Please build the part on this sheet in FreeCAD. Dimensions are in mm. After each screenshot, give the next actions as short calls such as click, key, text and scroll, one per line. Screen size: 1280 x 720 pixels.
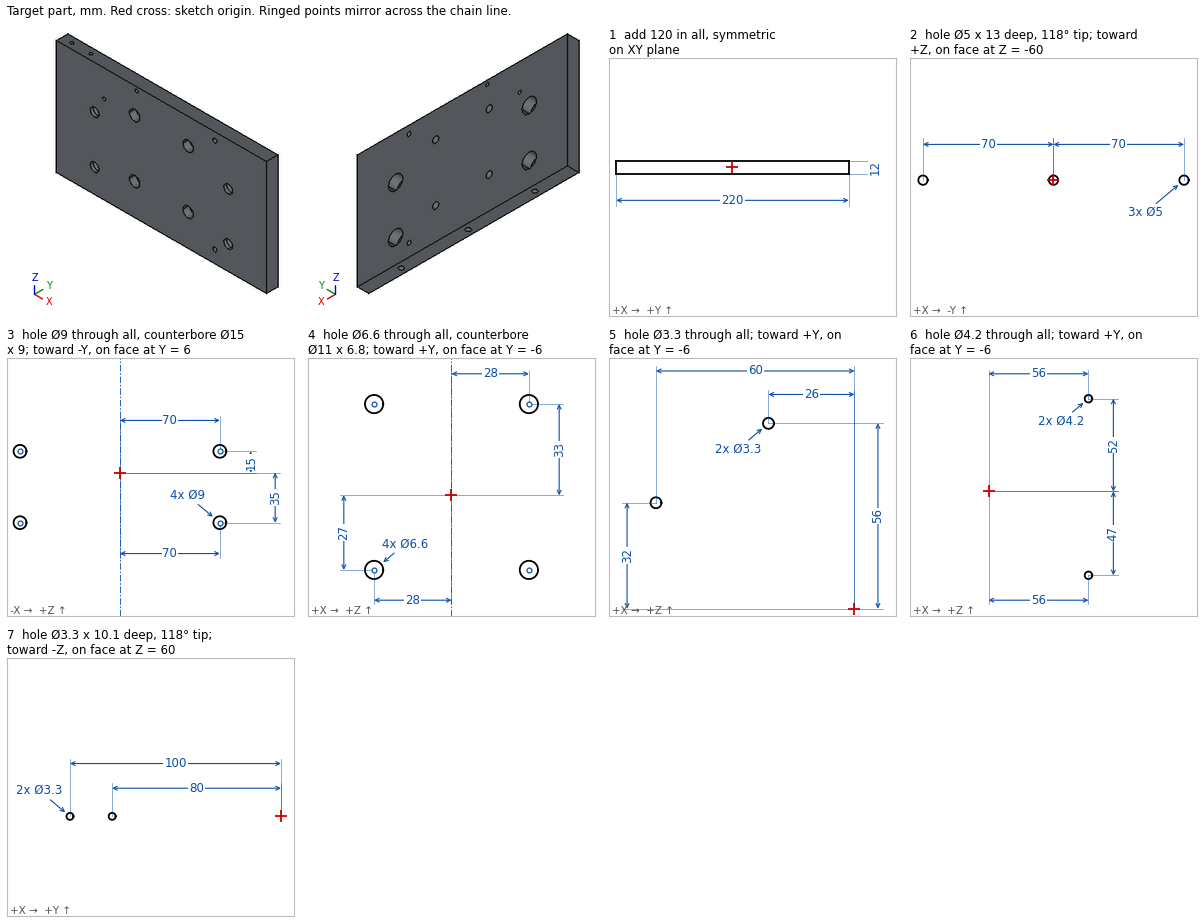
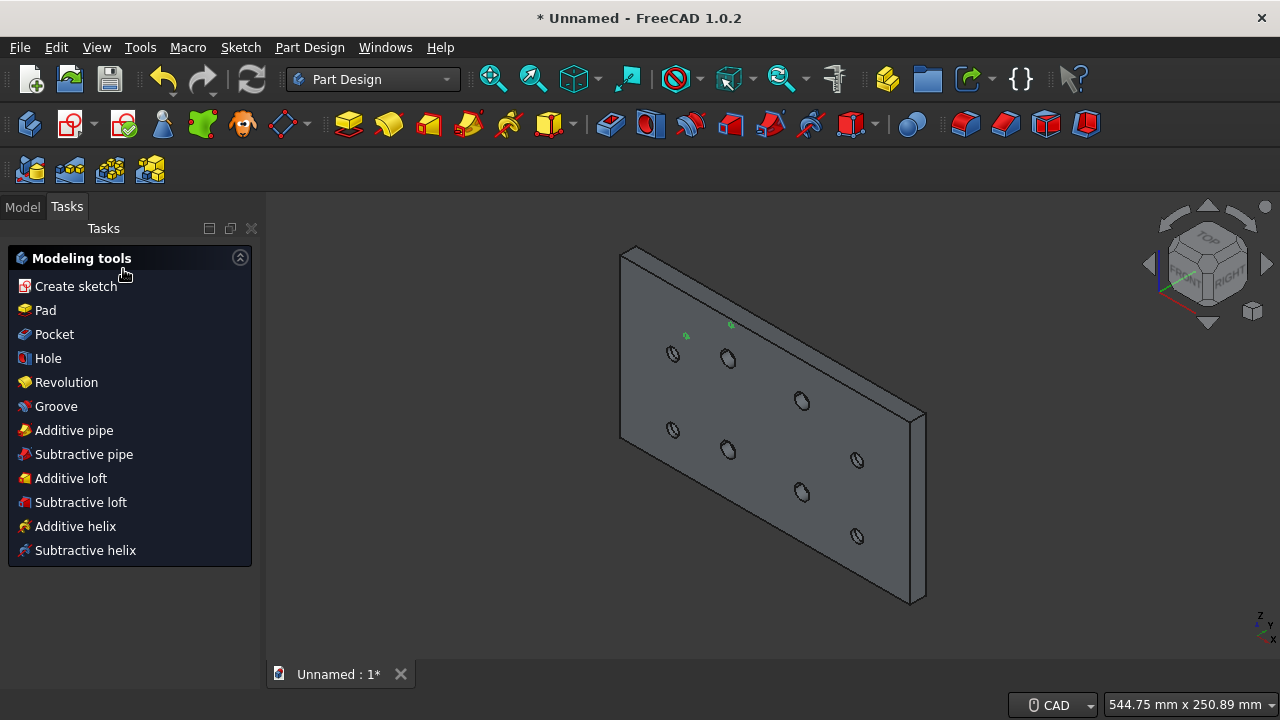
click(652, 124)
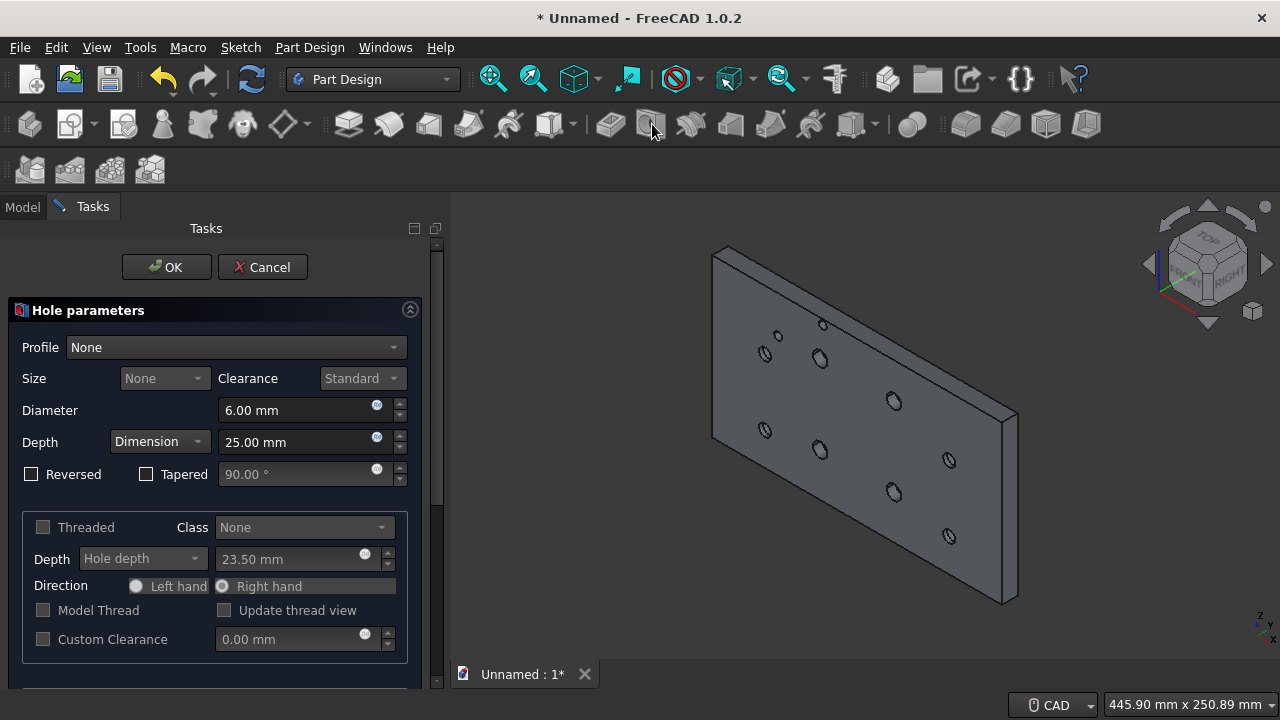
triple_click(305, 410)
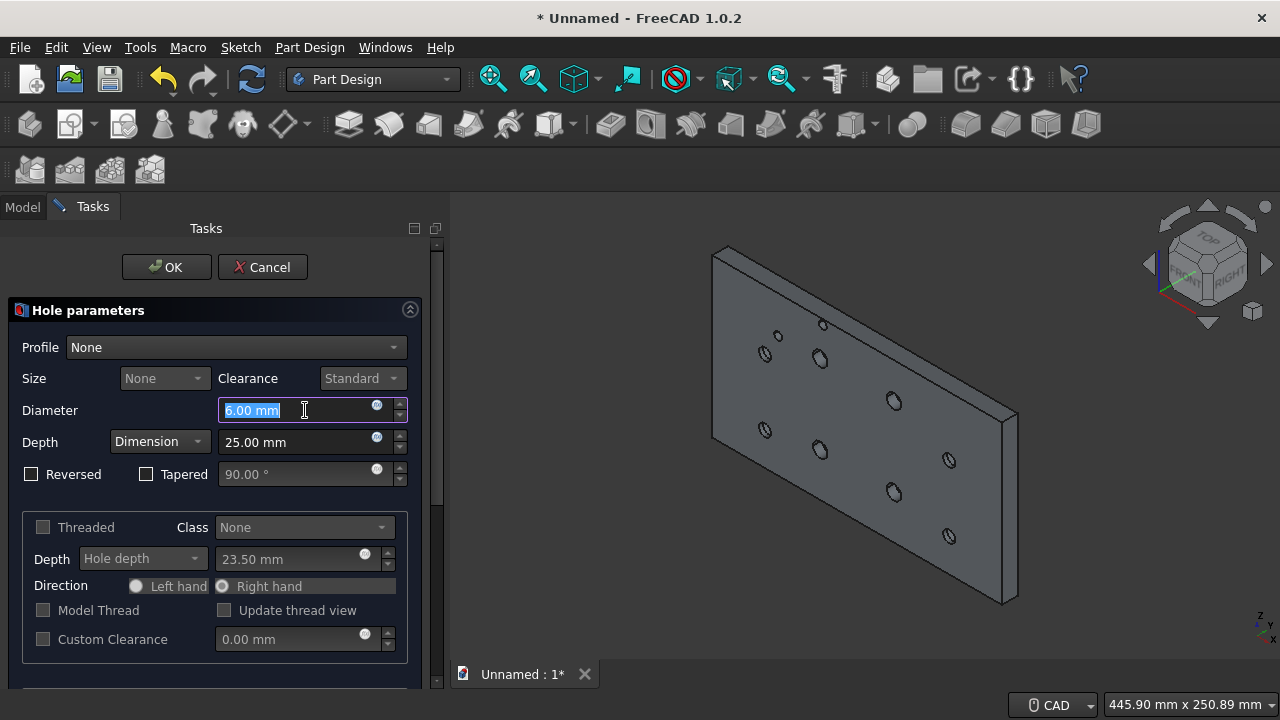
text(3.3)
key(Tab)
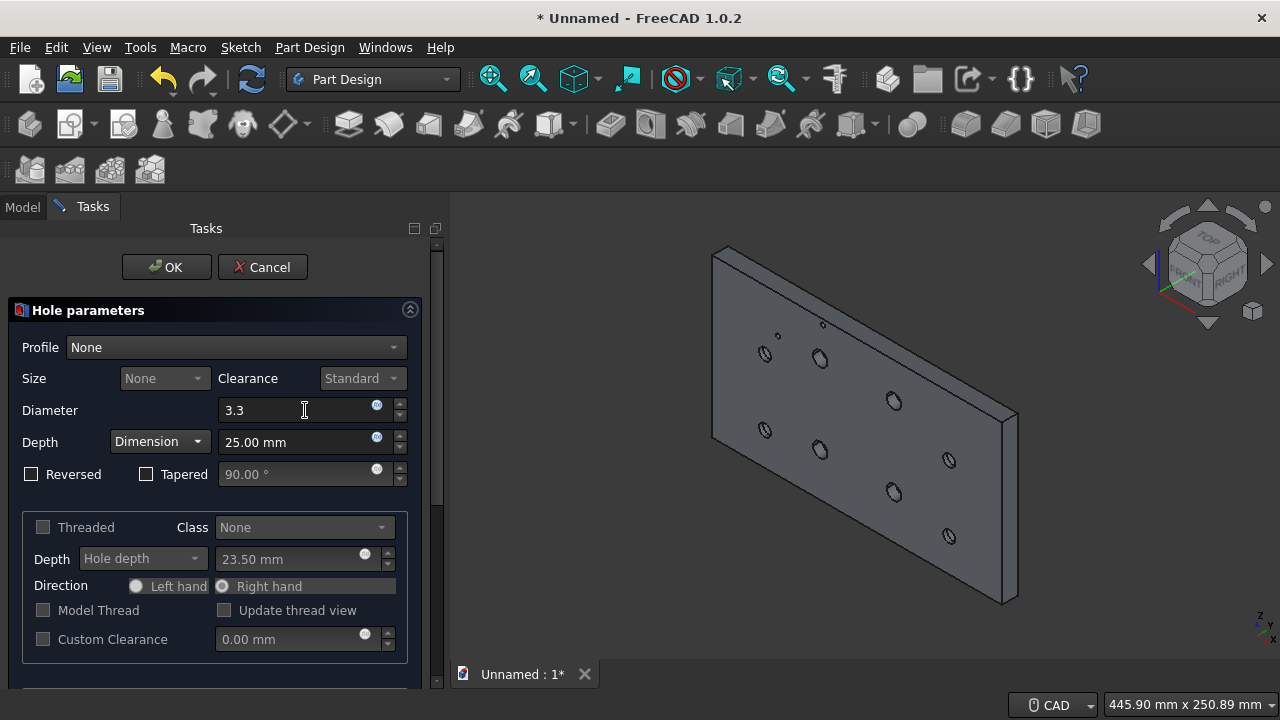
click(161, 442)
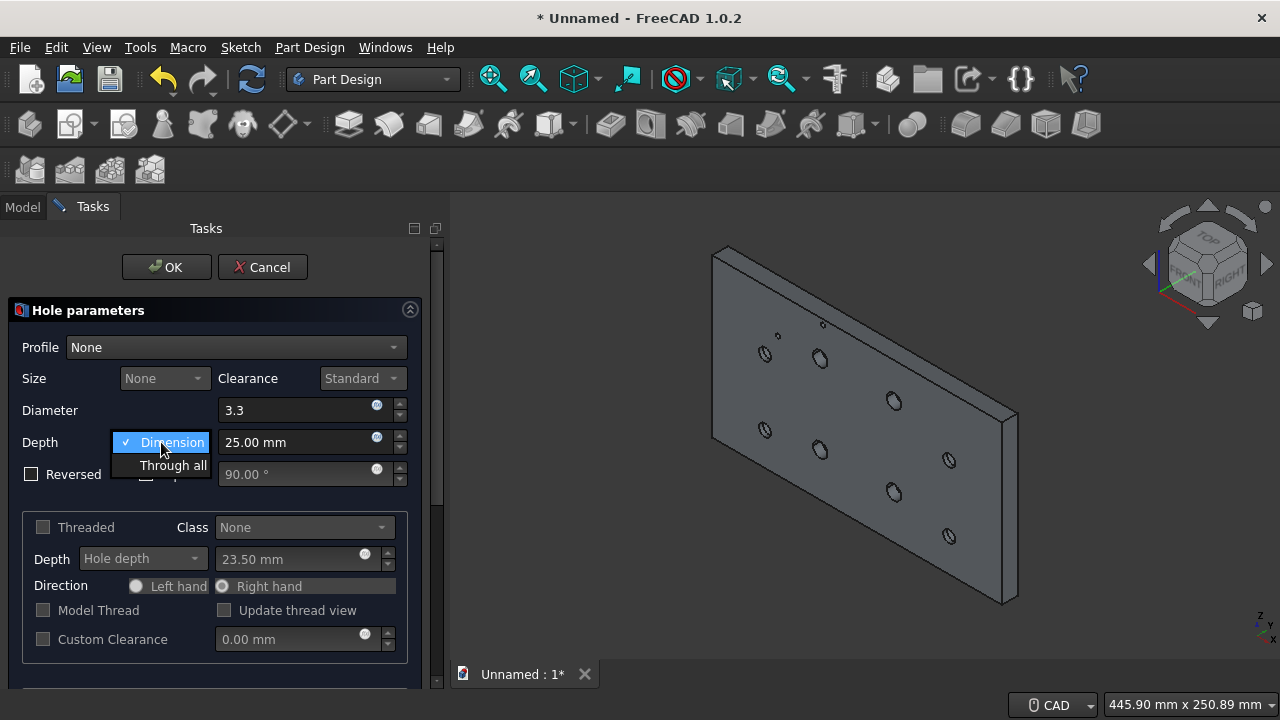
click(160, 466)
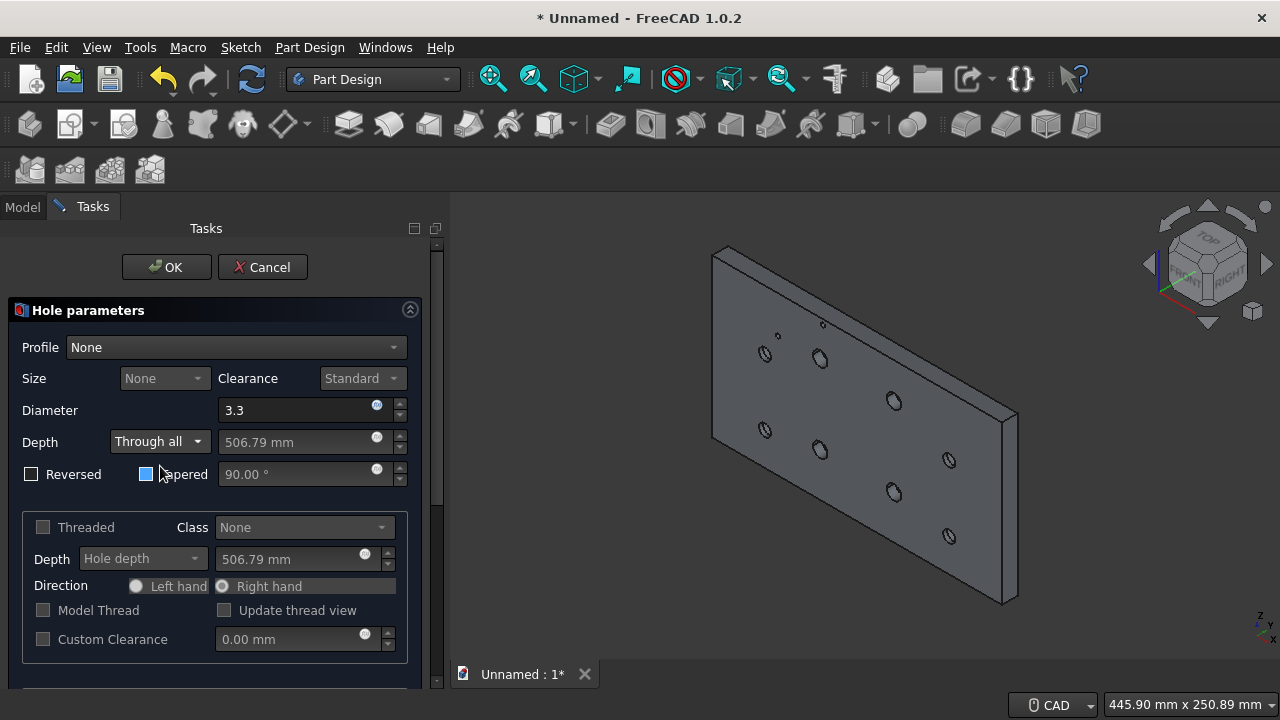
click(167, 267)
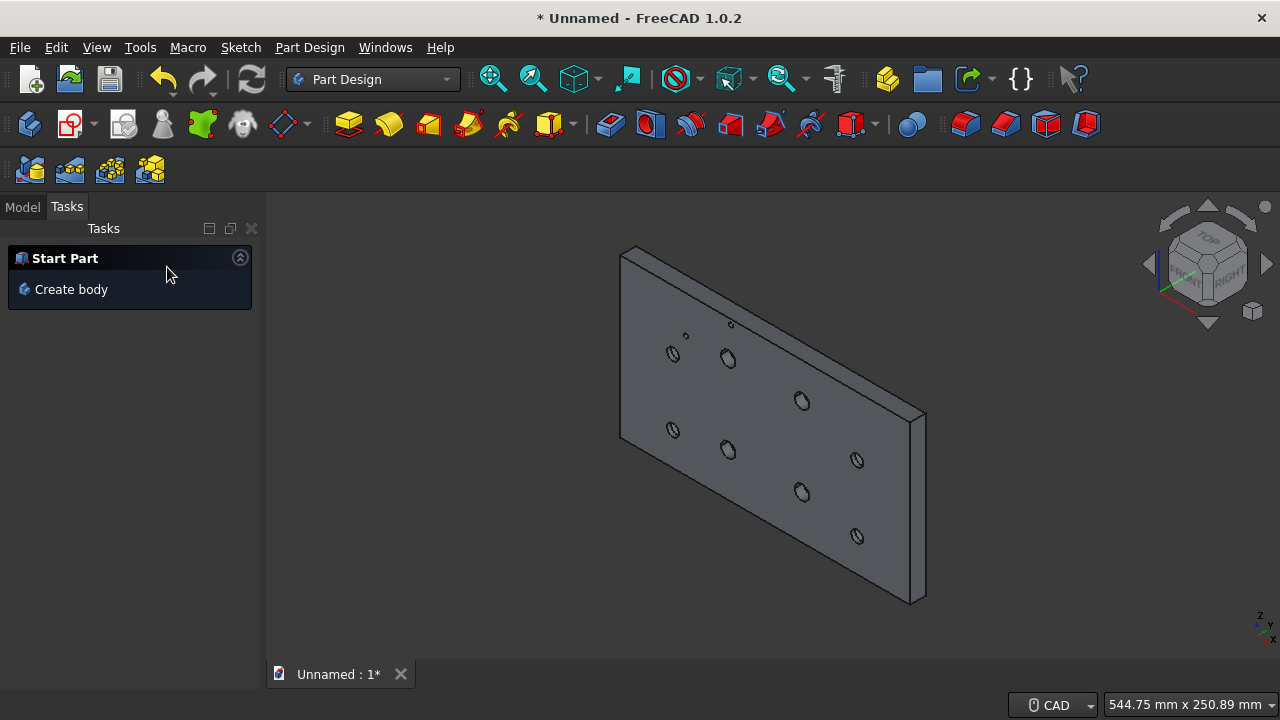
click(765, 429)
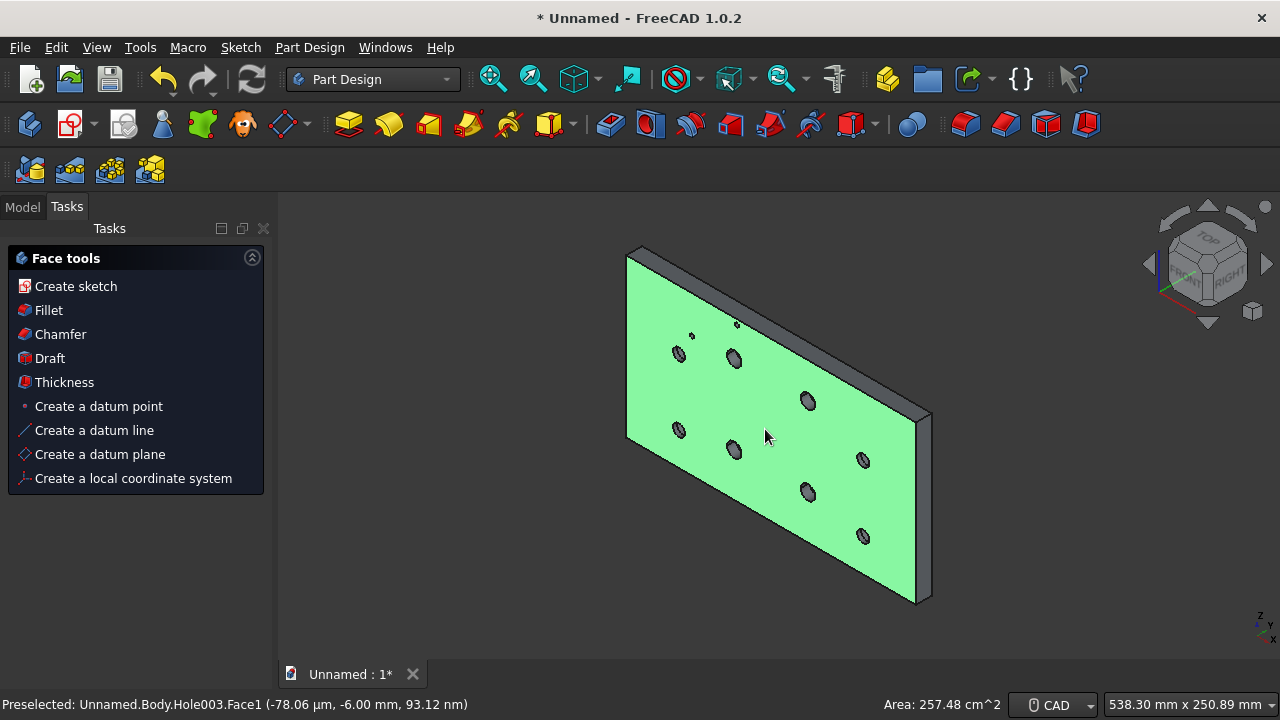
click(70, 124)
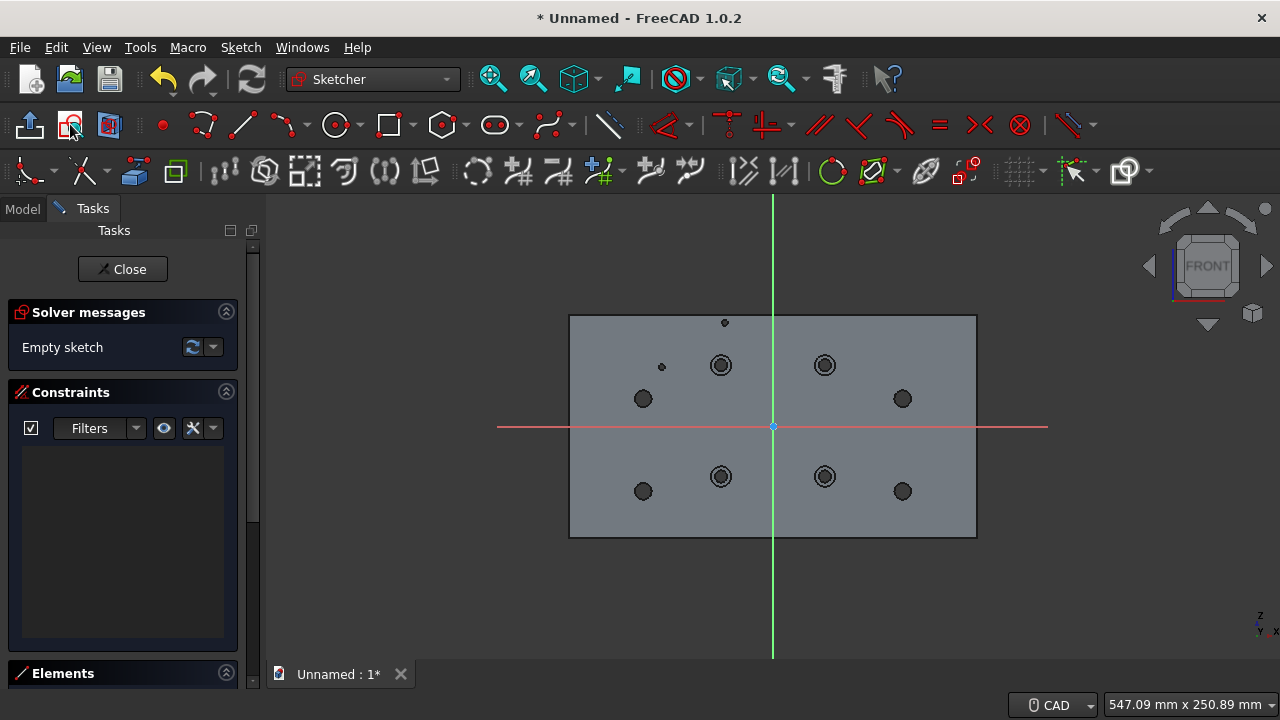
scroll(1076, 412, up, 2)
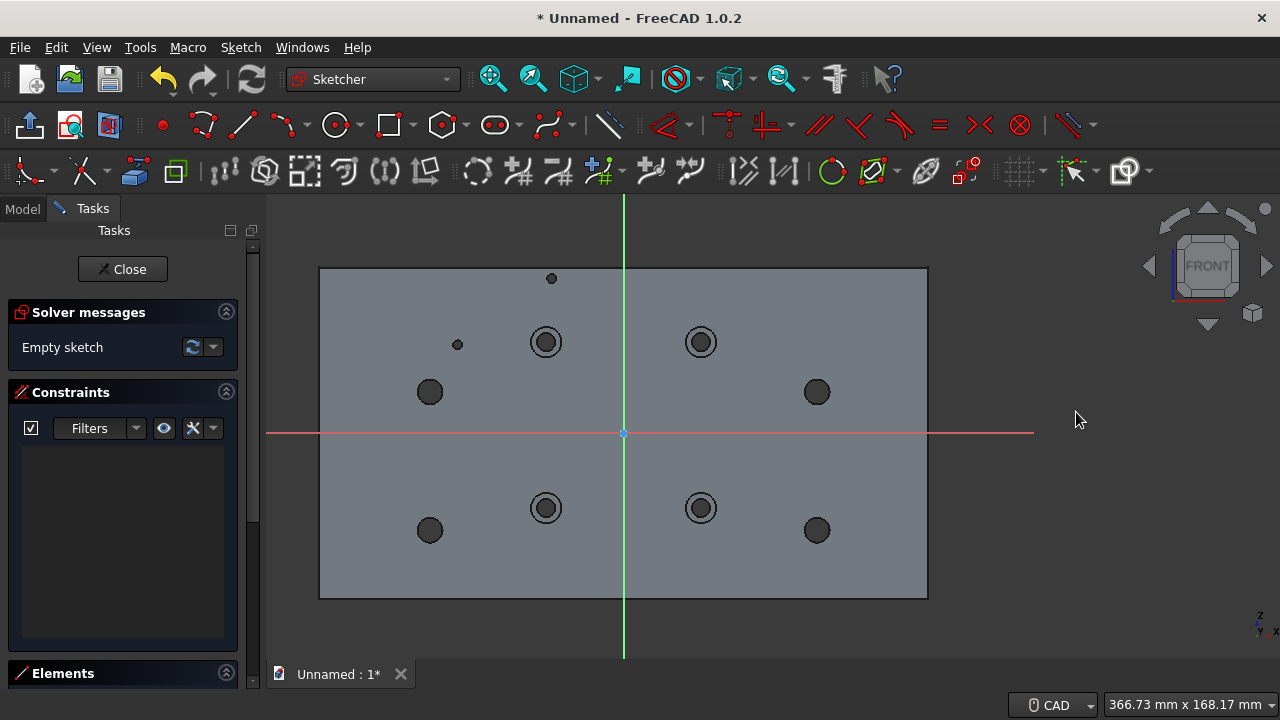
click(336, 126)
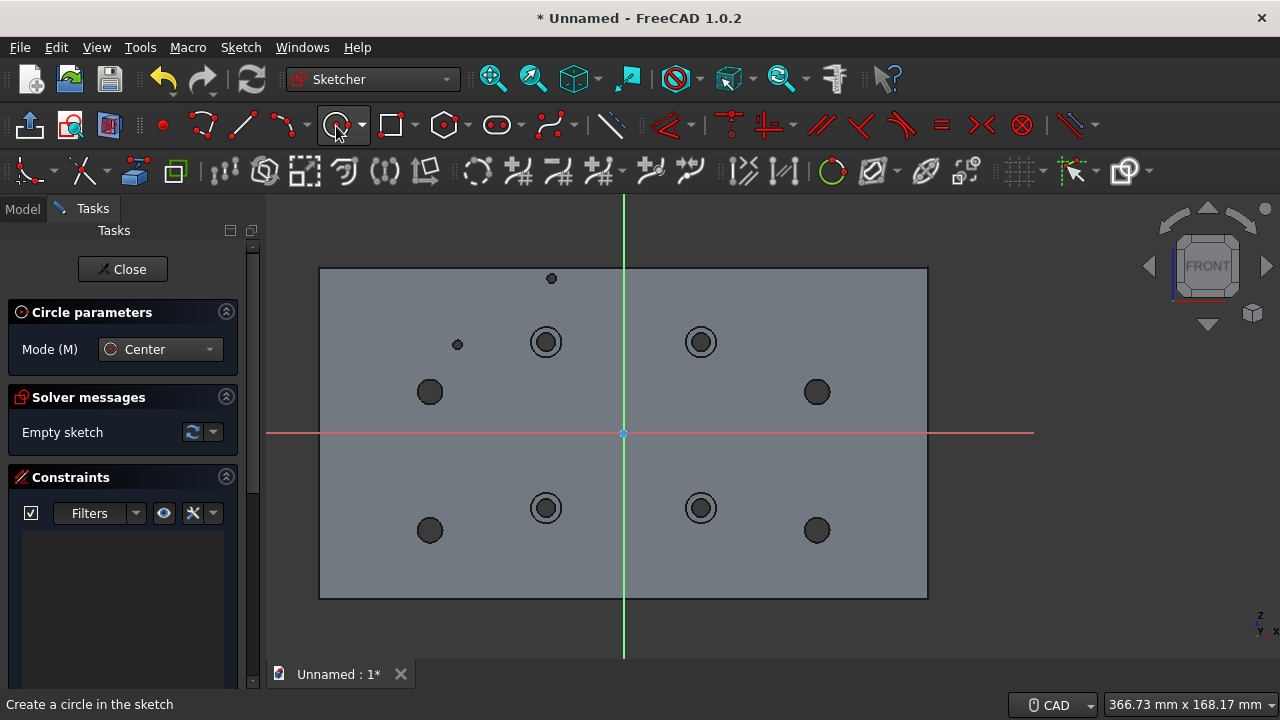
scroll(778, 290, up, 7)